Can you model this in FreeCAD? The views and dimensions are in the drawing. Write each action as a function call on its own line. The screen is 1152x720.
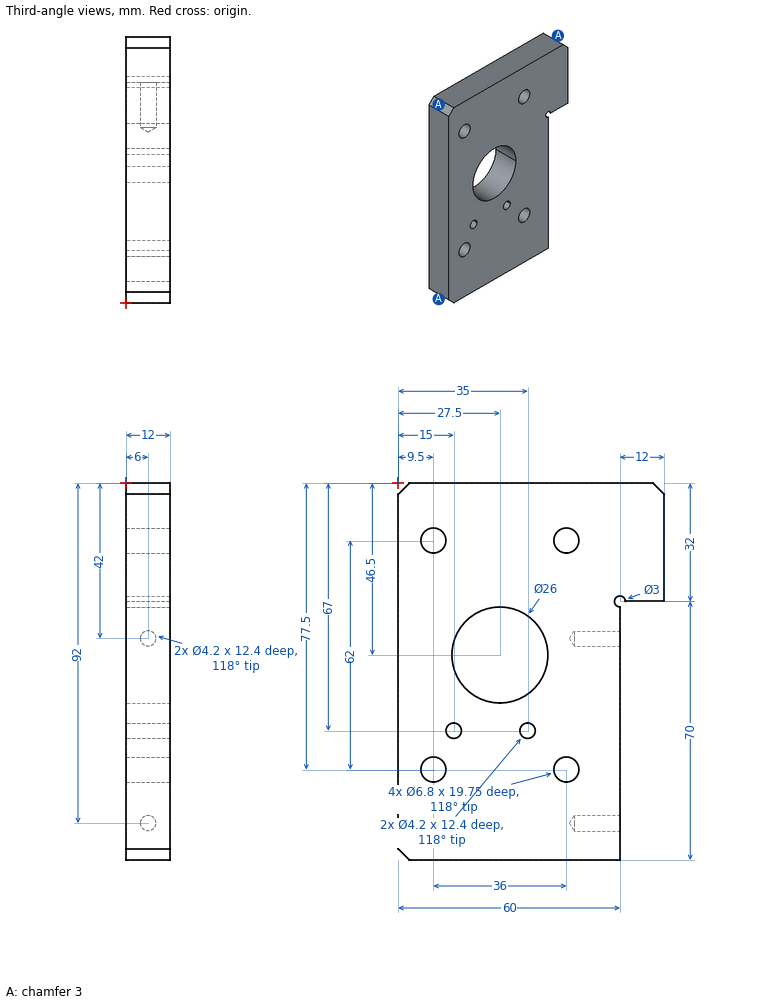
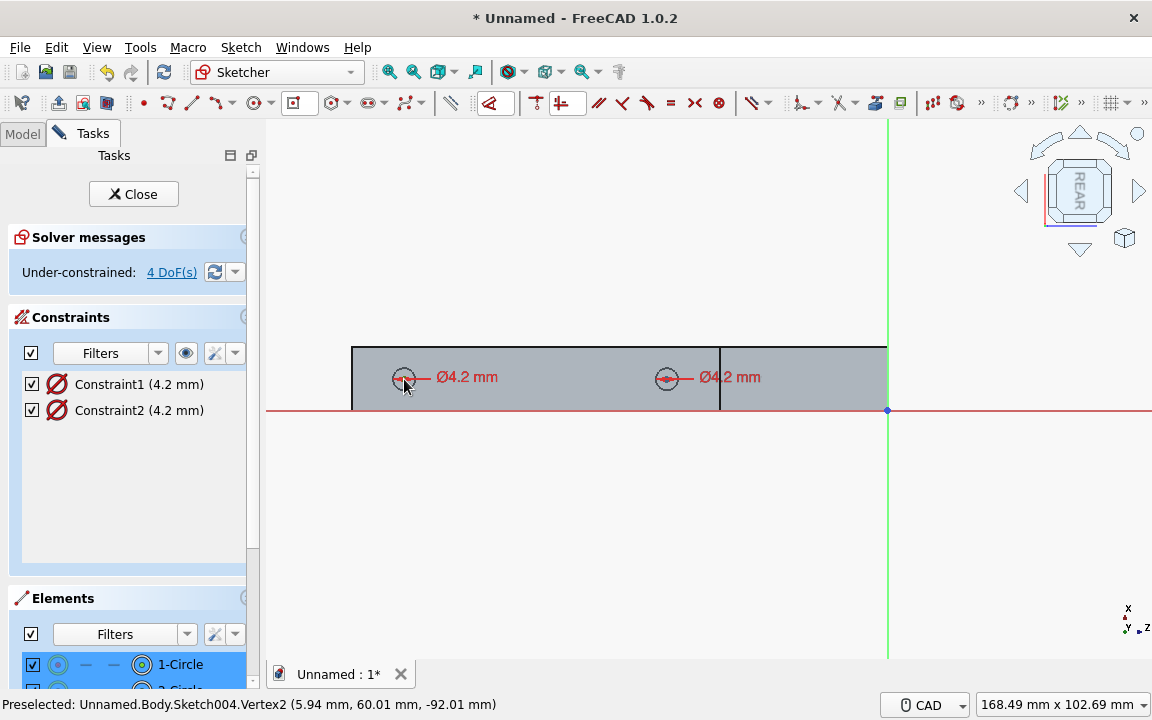
click(580, 104)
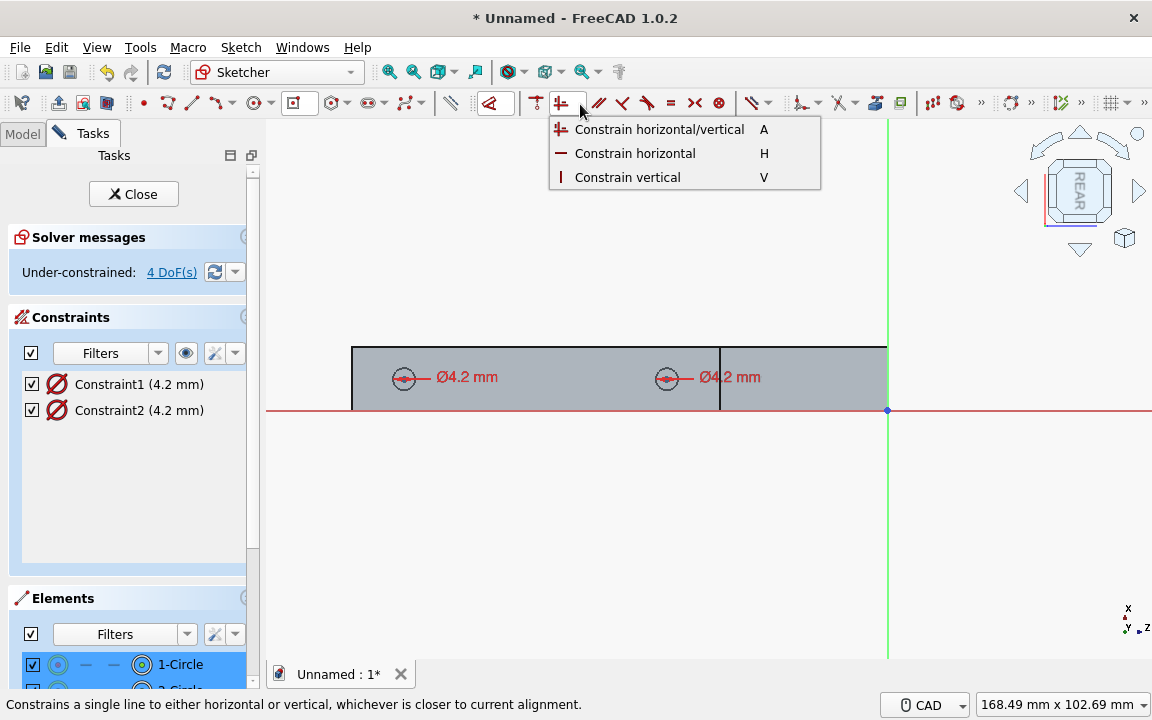
click(685, 153)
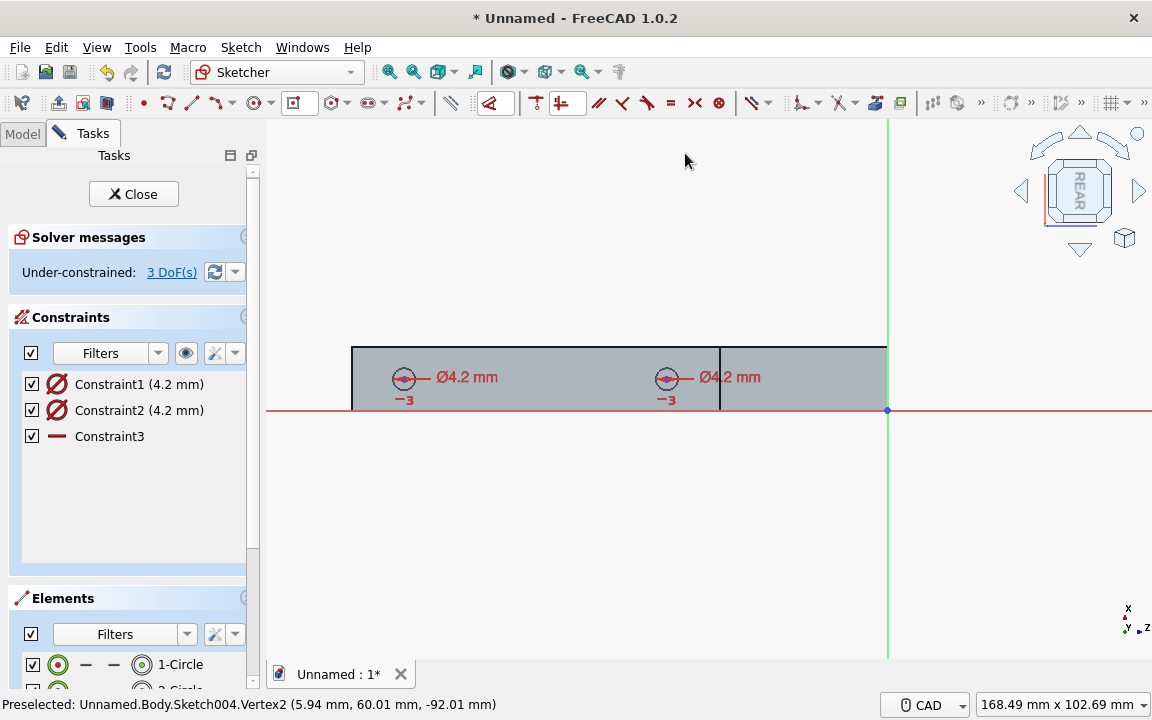
scroll(667, 379, up, 2)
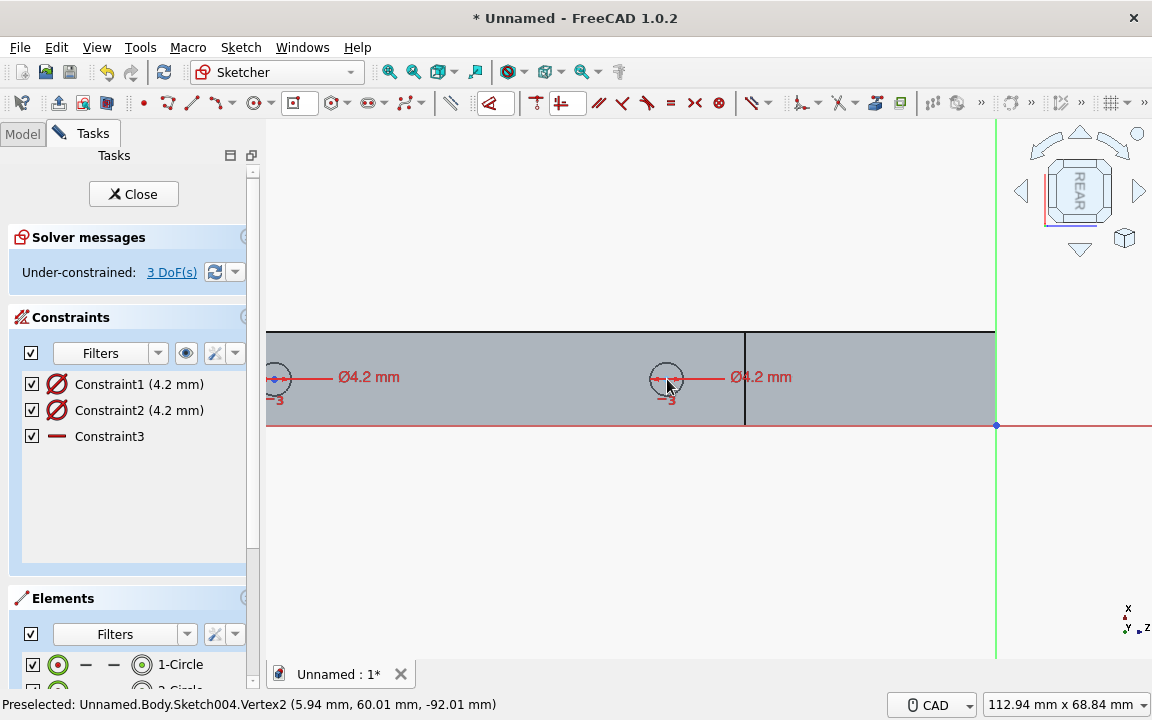
click(667, 379)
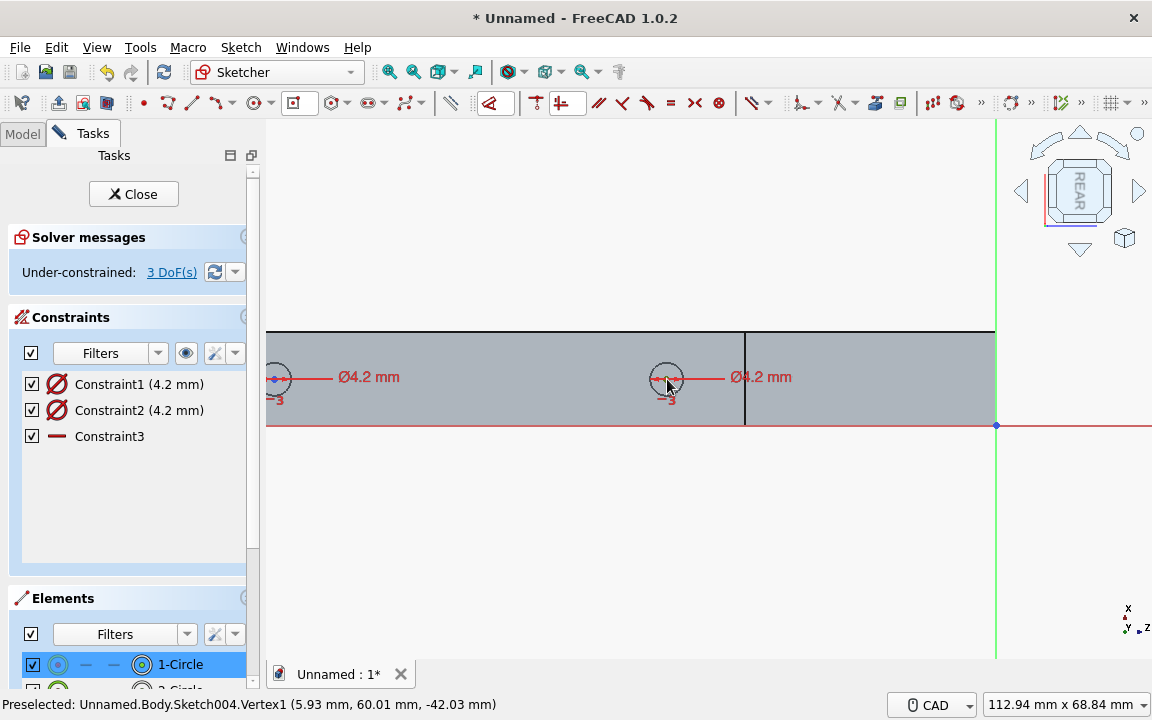
click(508, 104)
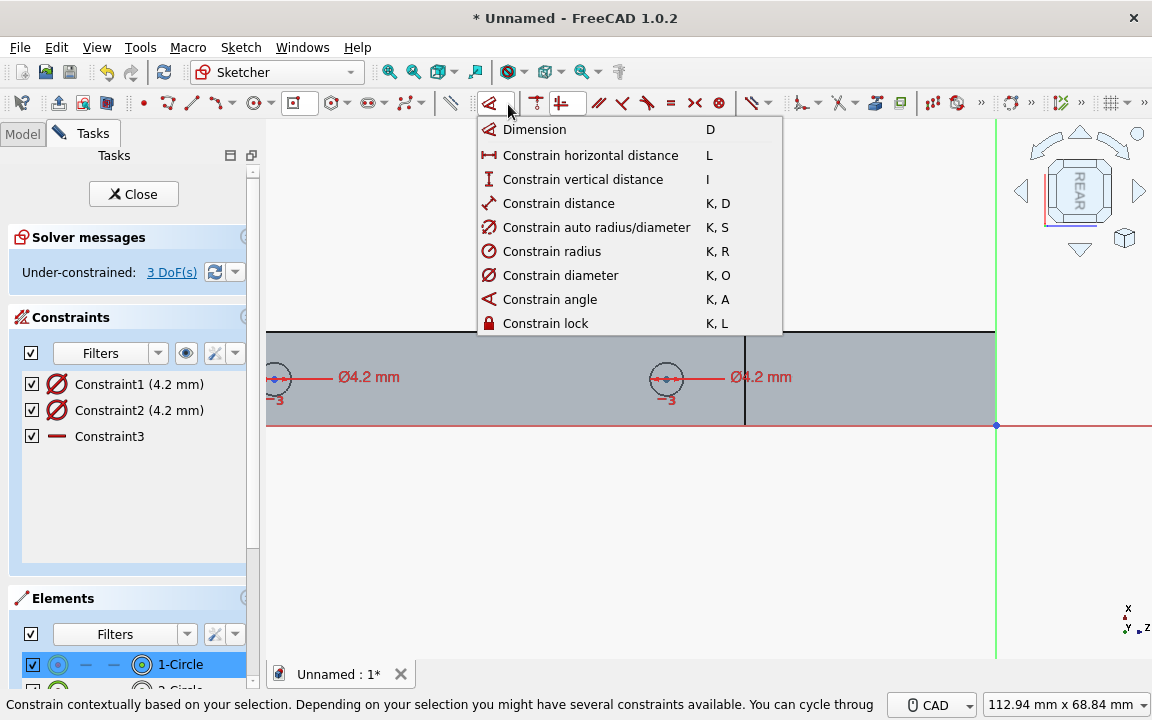
click(630, 179)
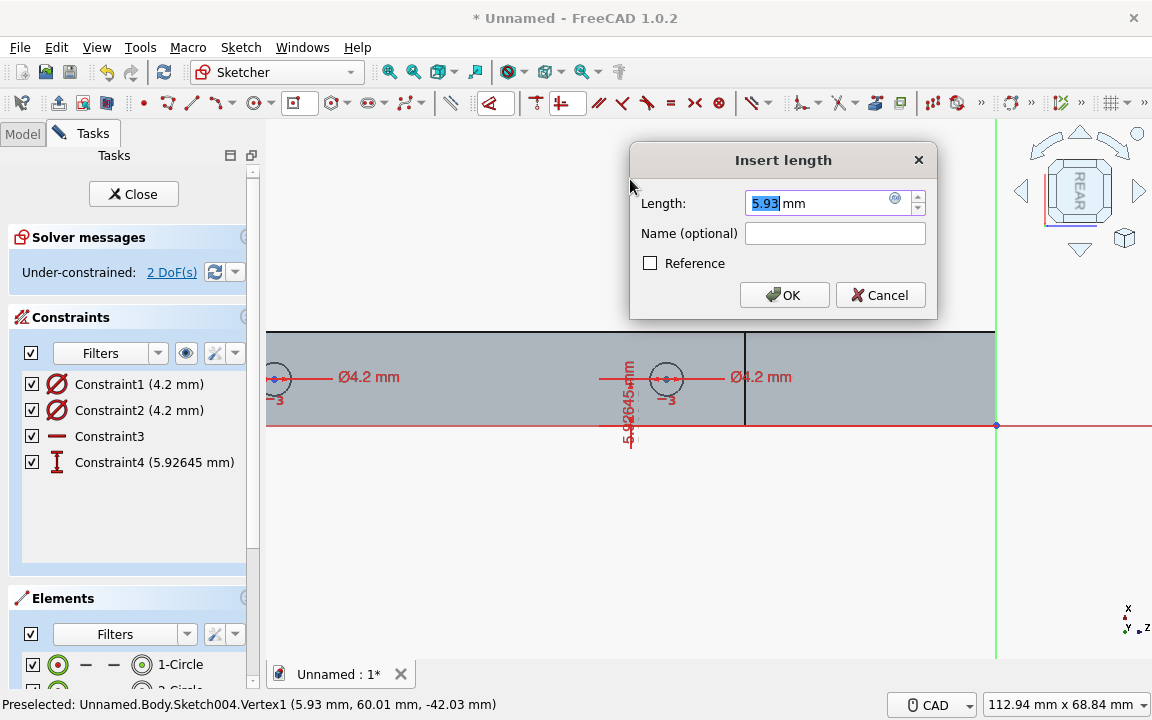
text(6)
key(Return)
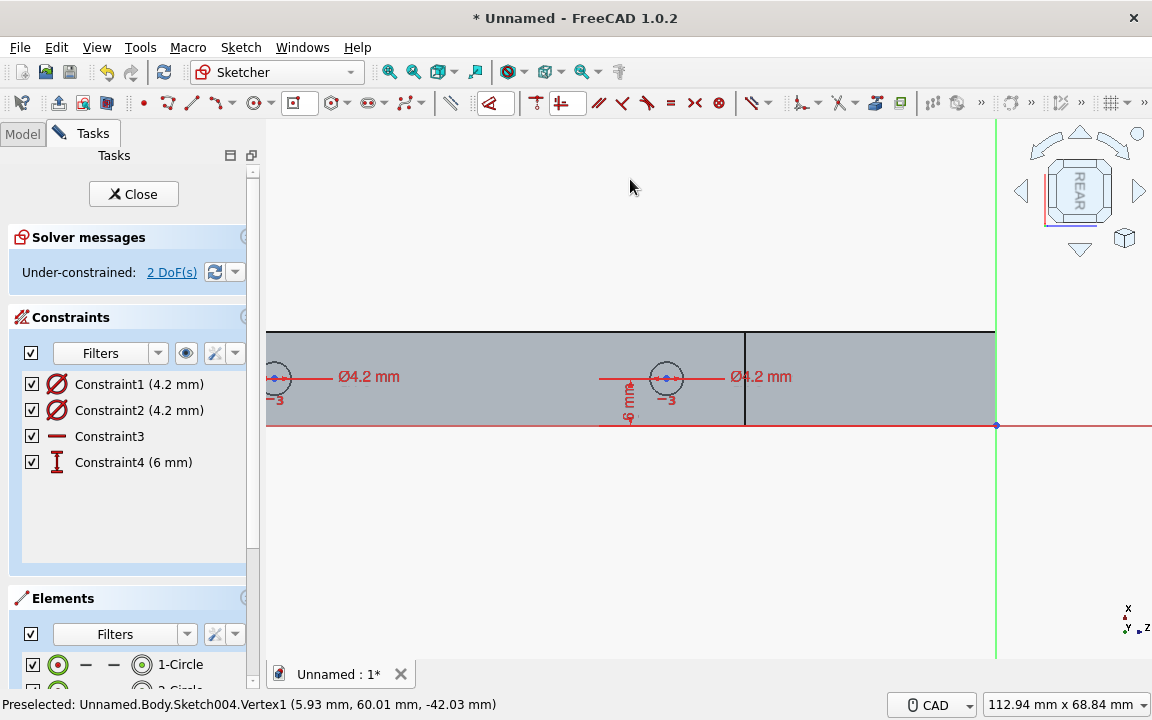
click(667, 379)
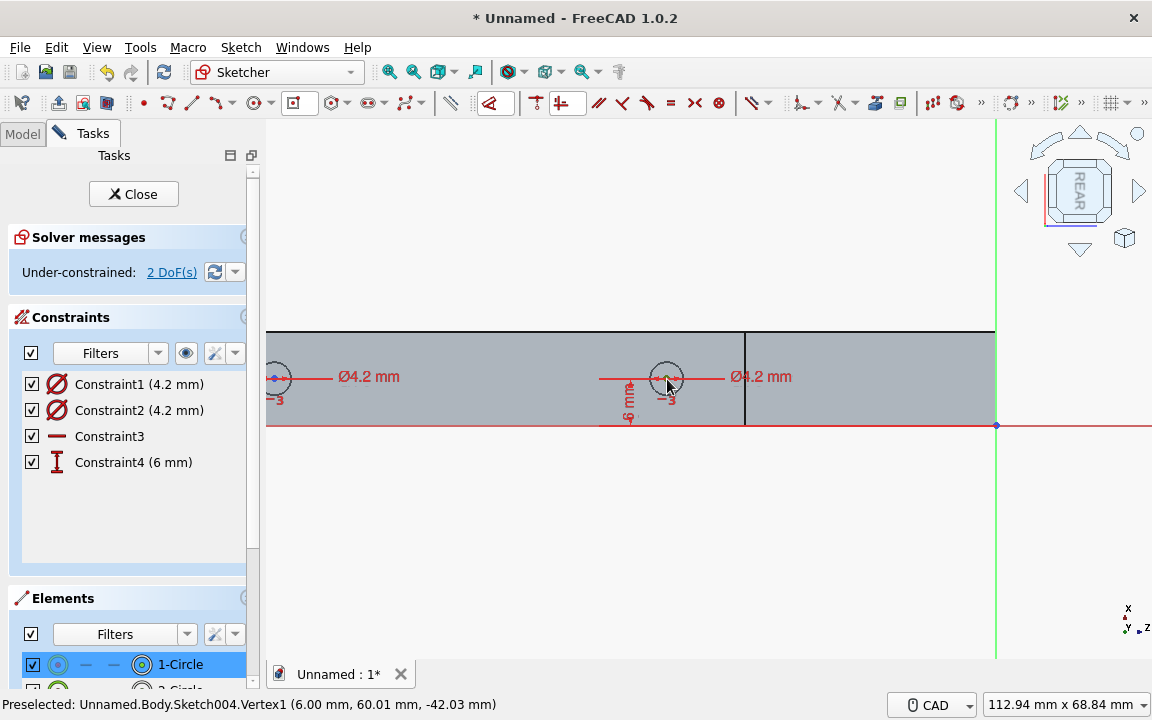
click(508, 104)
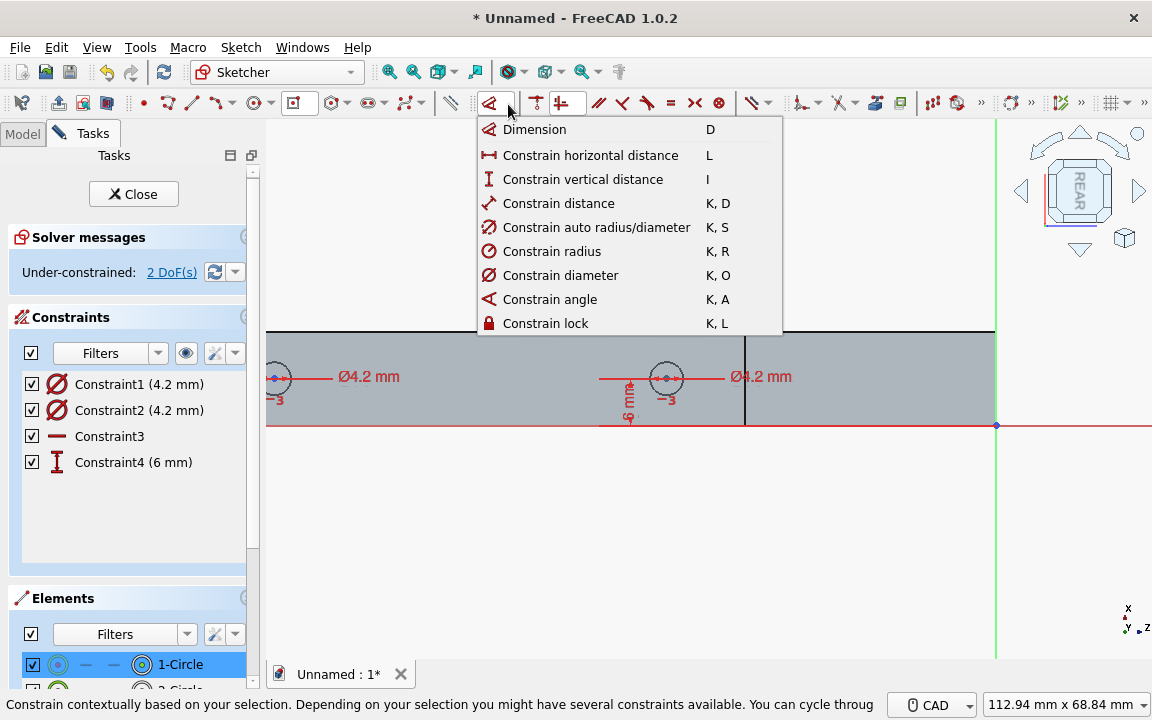
click(630, 155)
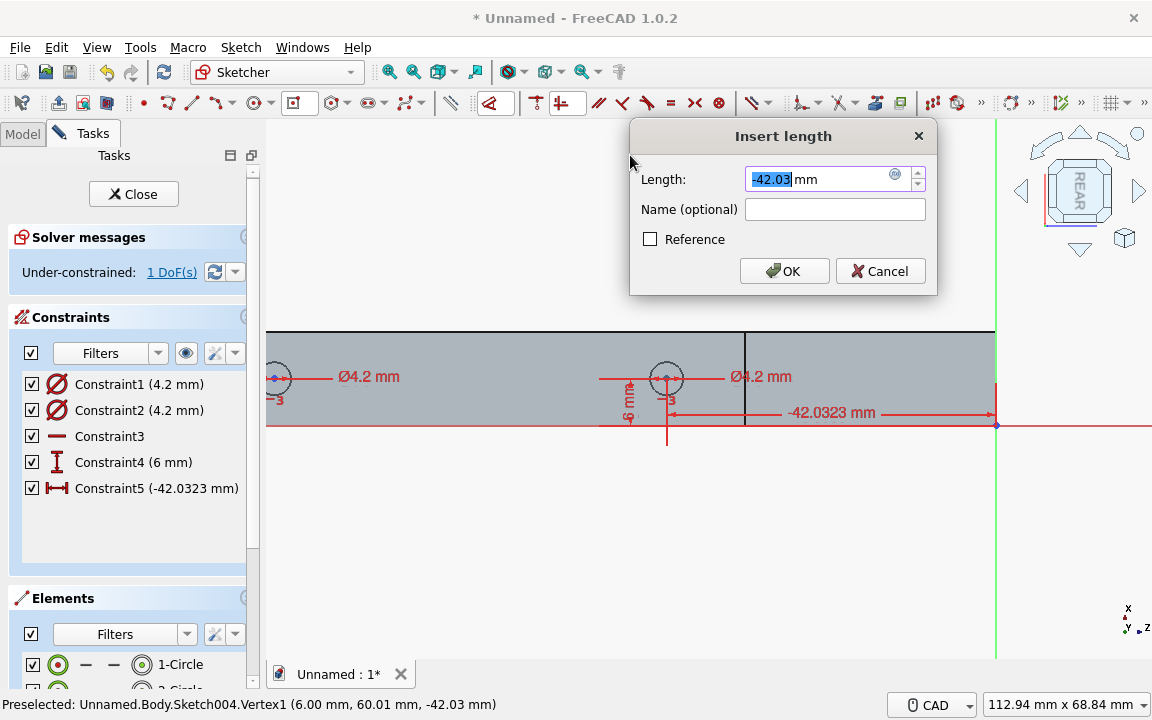
text(-42)
key(Return)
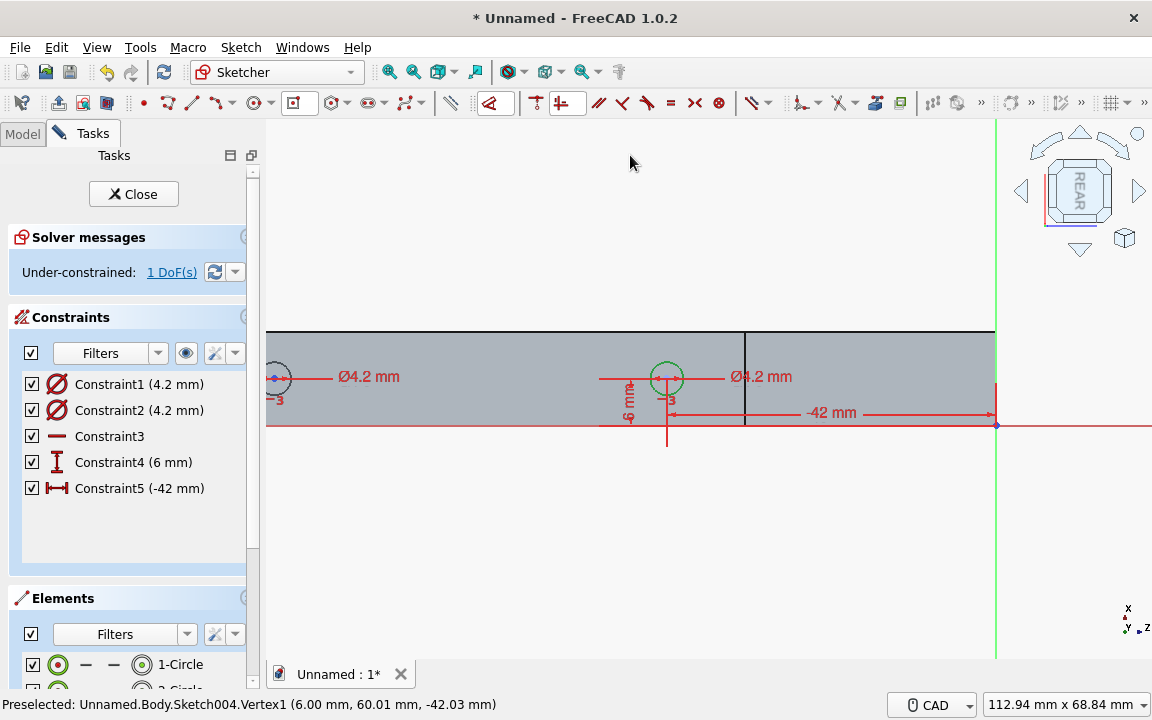
scroll(667, 379, down, 2)